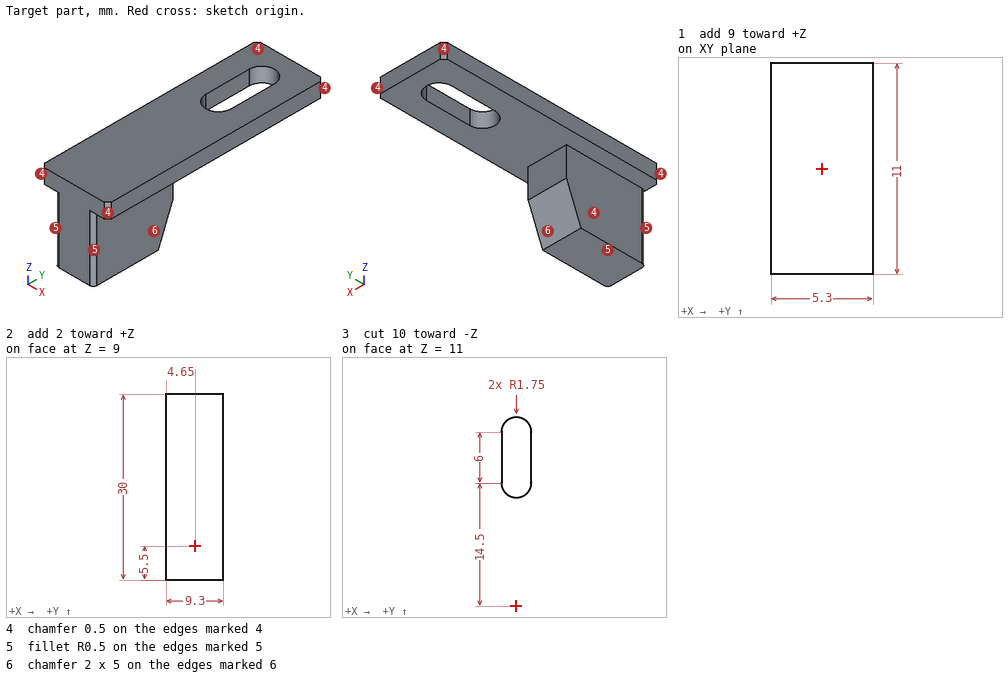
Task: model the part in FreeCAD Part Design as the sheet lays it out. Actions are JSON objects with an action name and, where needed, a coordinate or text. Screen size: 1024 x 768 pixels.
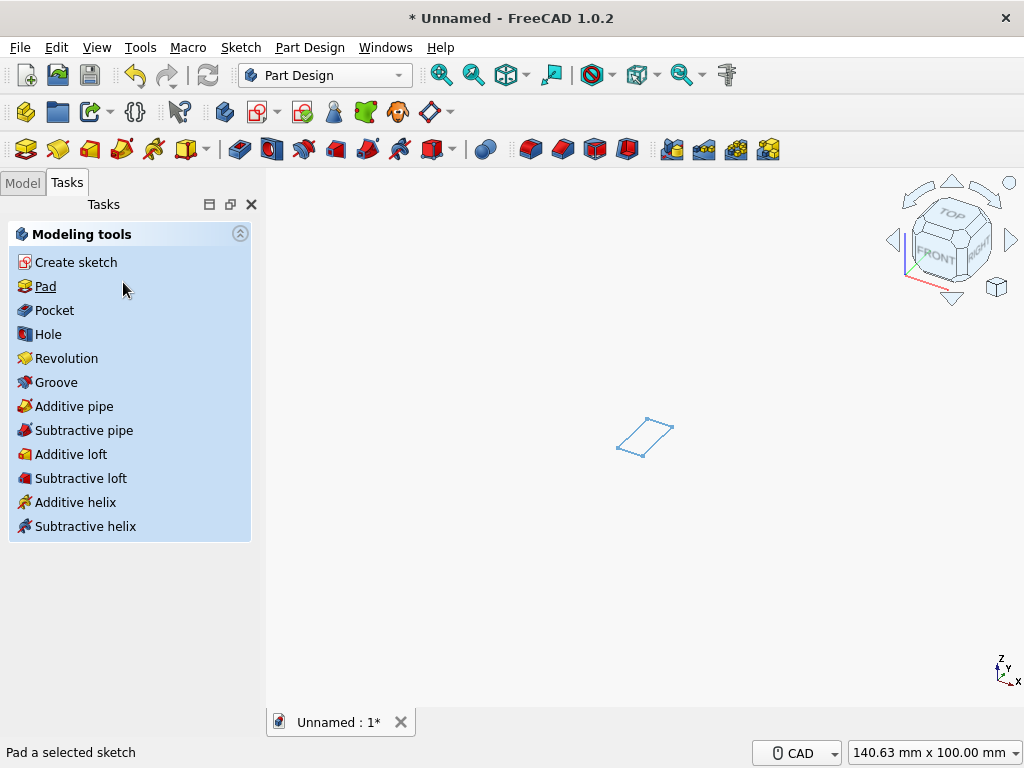
{"action": "left_click", "coordinate": [26, 150]}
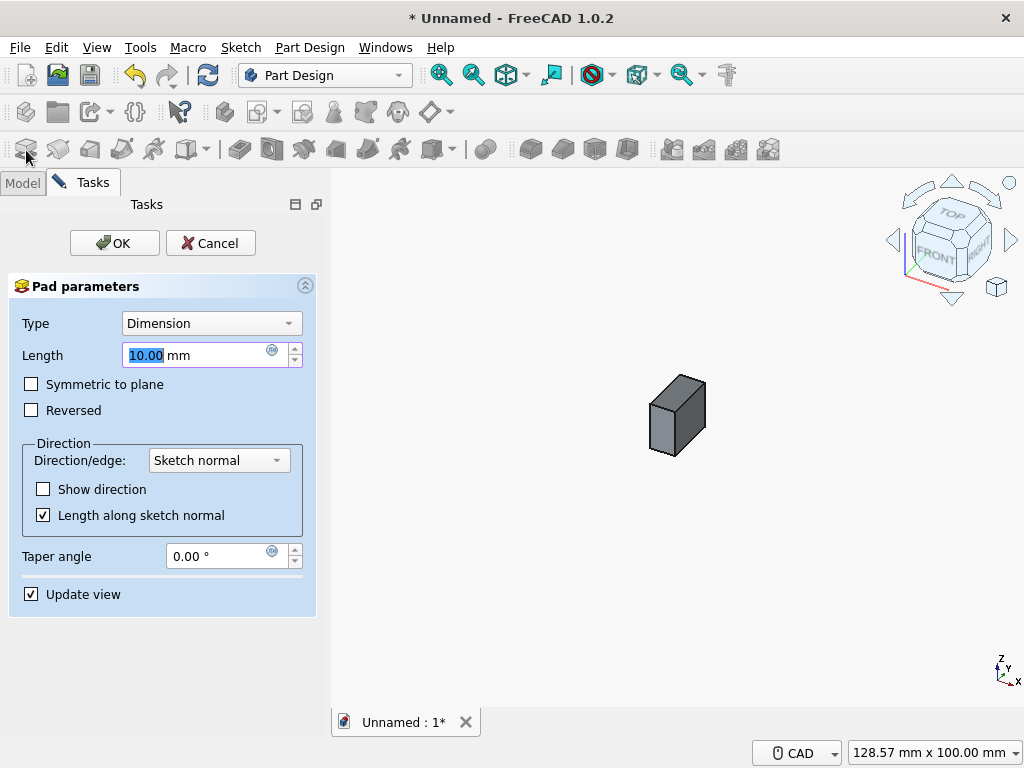
{"action": "type", "text": "9"}
{"action": "key", "text": "Tab"}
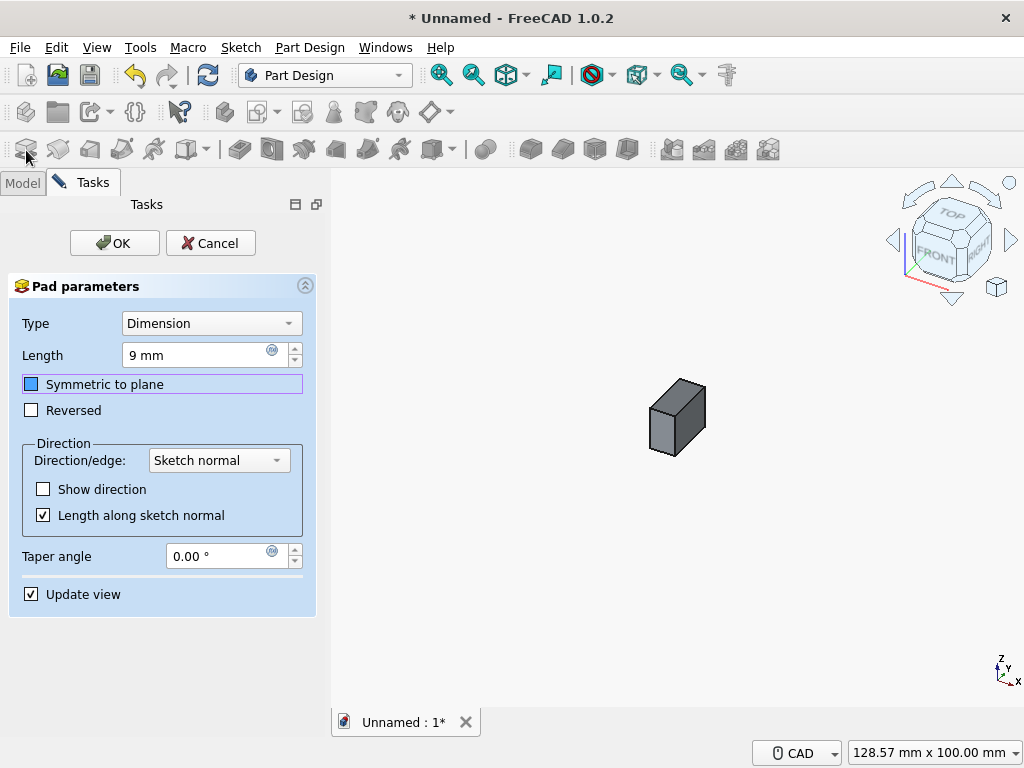
{"action": "left_click", "coordinate": [115, 243]}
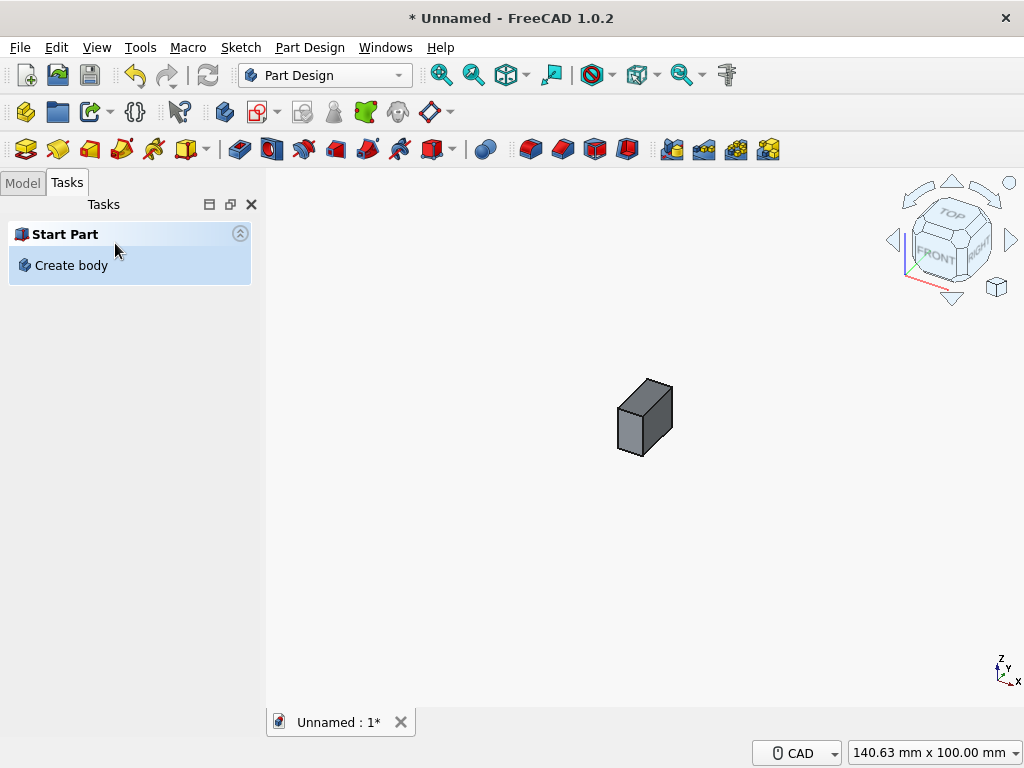
{"action": "left_click", "coordinate": [442, 76]}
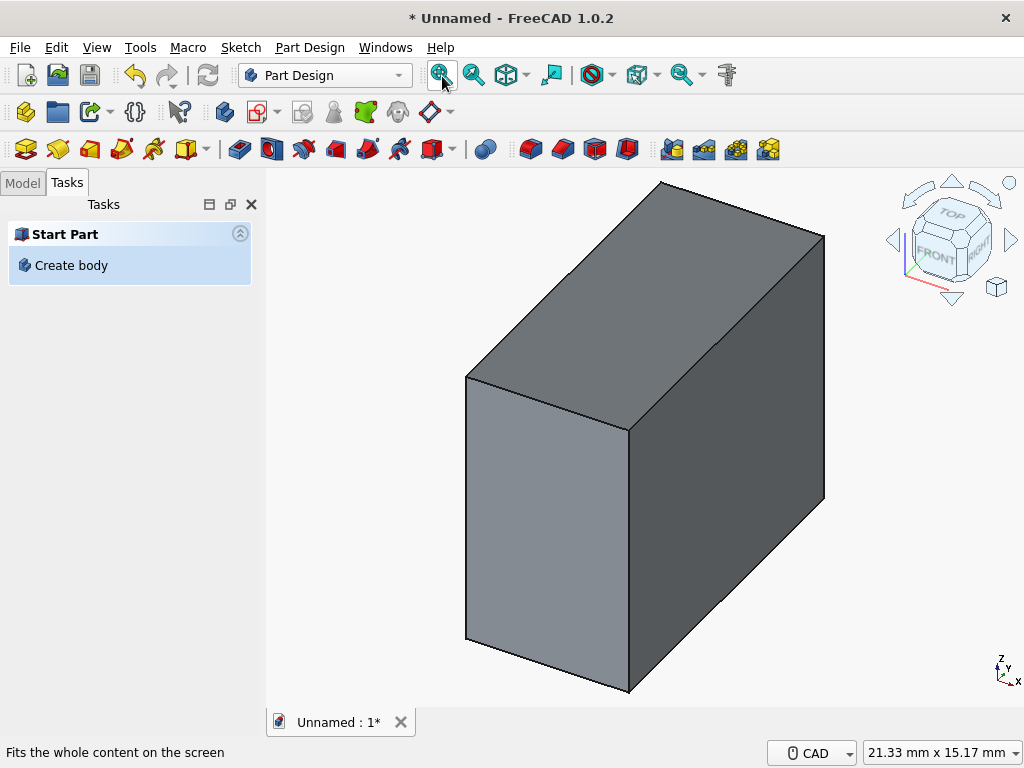
{"action": "left_click", "coordinate": [673, 278]}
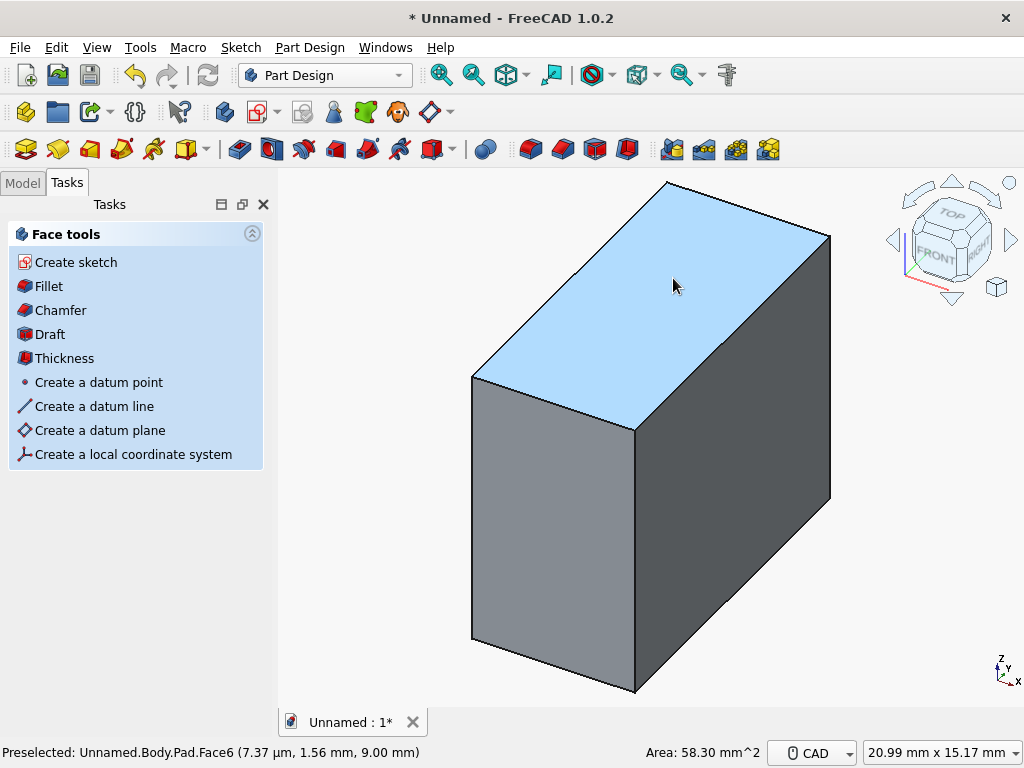
{"action": "left_click", "coordinate": [258, 112]}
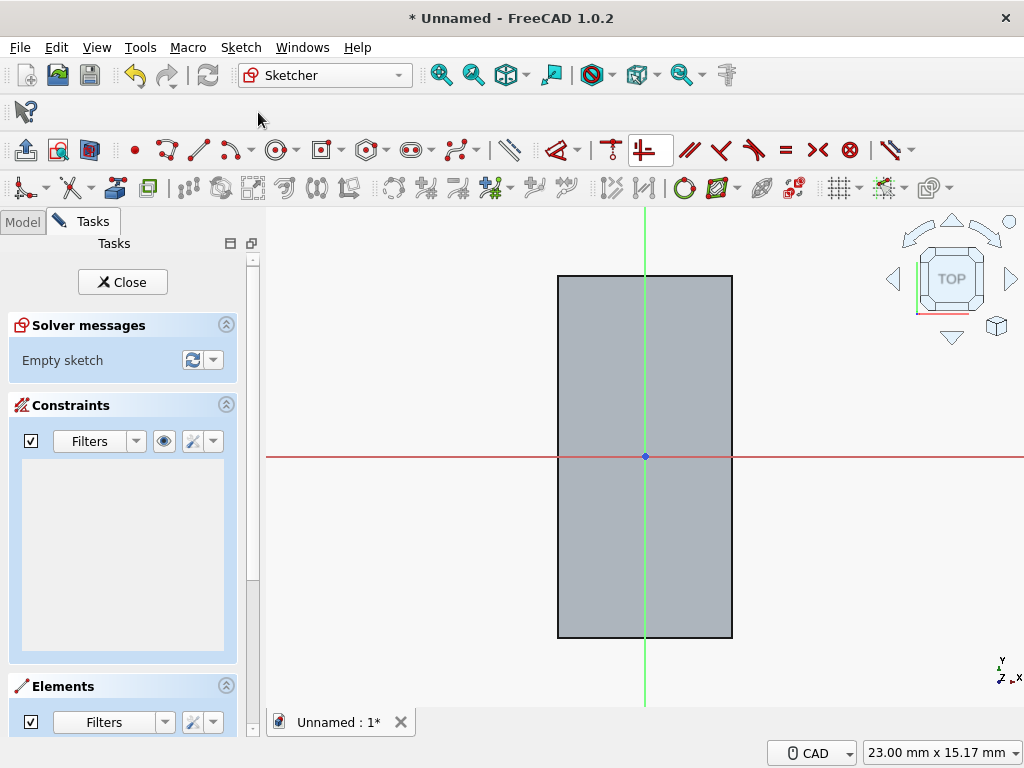
{"action": "scroll", "coordinate": [547, 592], "scroll_direction": "down", "scroll_amount": 6}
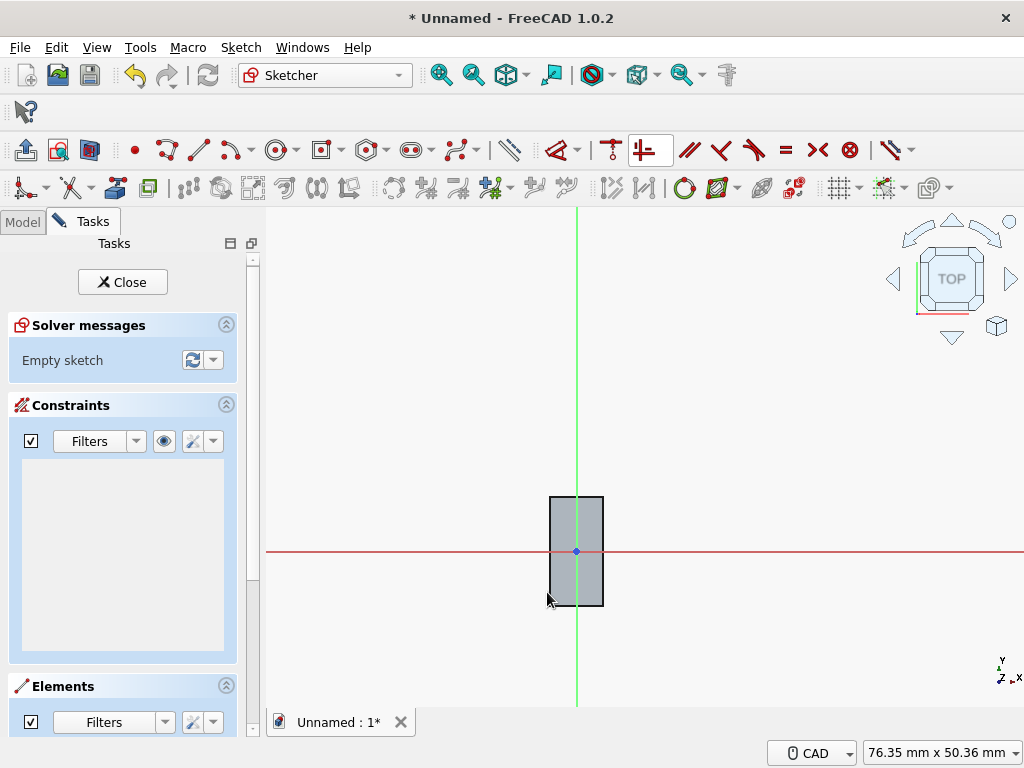
{"action": "key", "text": "g r"}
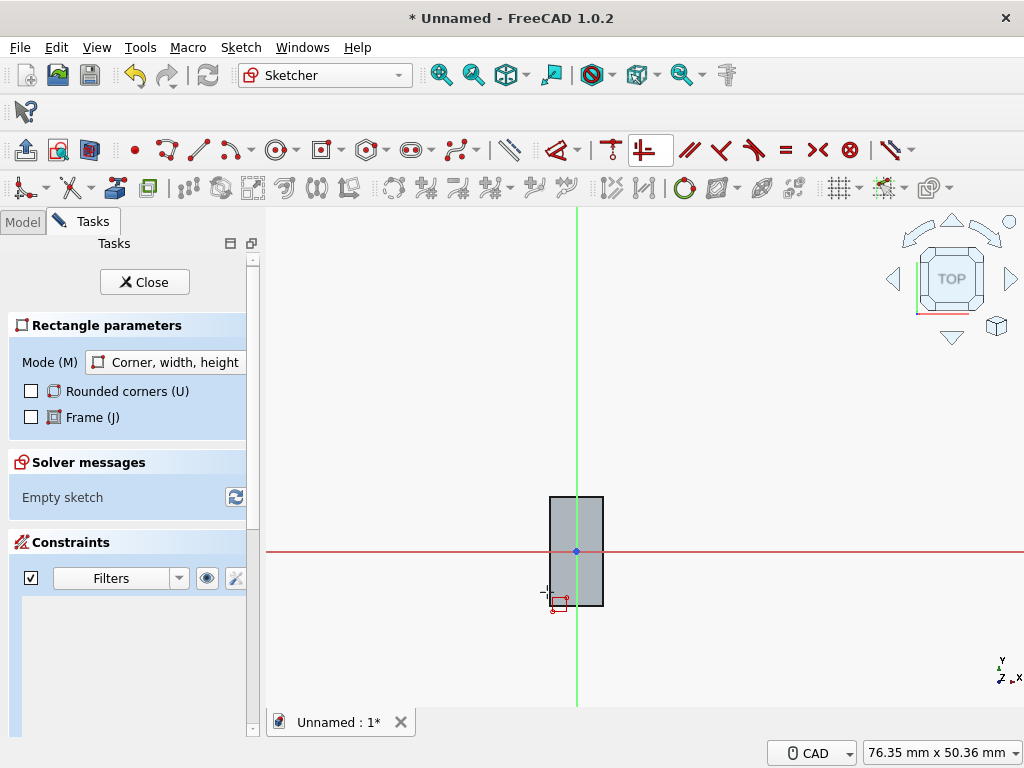
{"action": "left_click", "coordinate": [531, 309]}
{"action": "left_click", "coordinate": [623, 606]}
{"action": "key", "text": "Escape"}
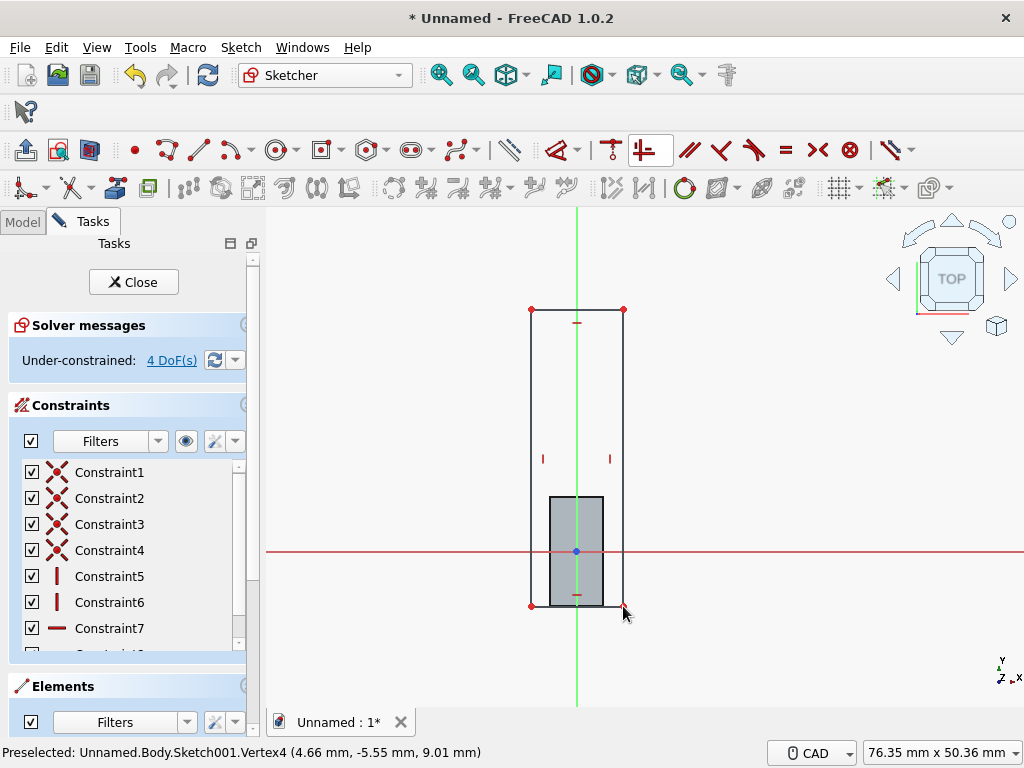
{"action": "left_click", "coordinate": [556, 150]}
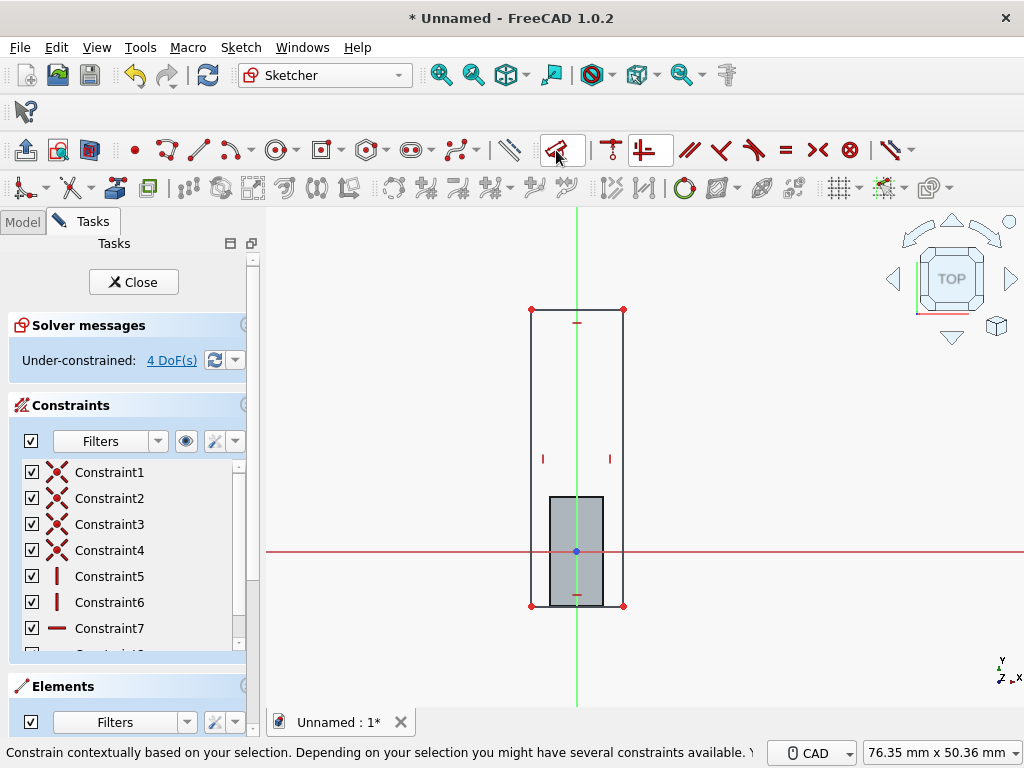
{"action": "left_click", "coordinate": [531, 399]}
{"action": "left_click", "coordinate": [497, 458]}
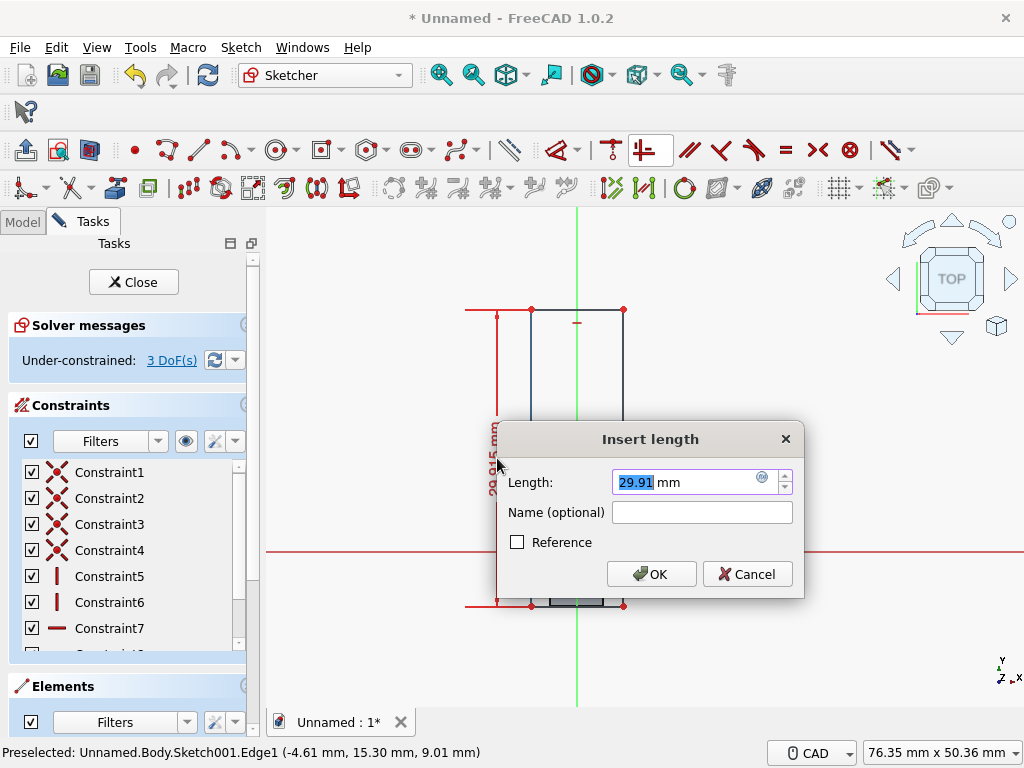
{"action": "type", "text": "30"}
{"action": "key", "text": "Return"}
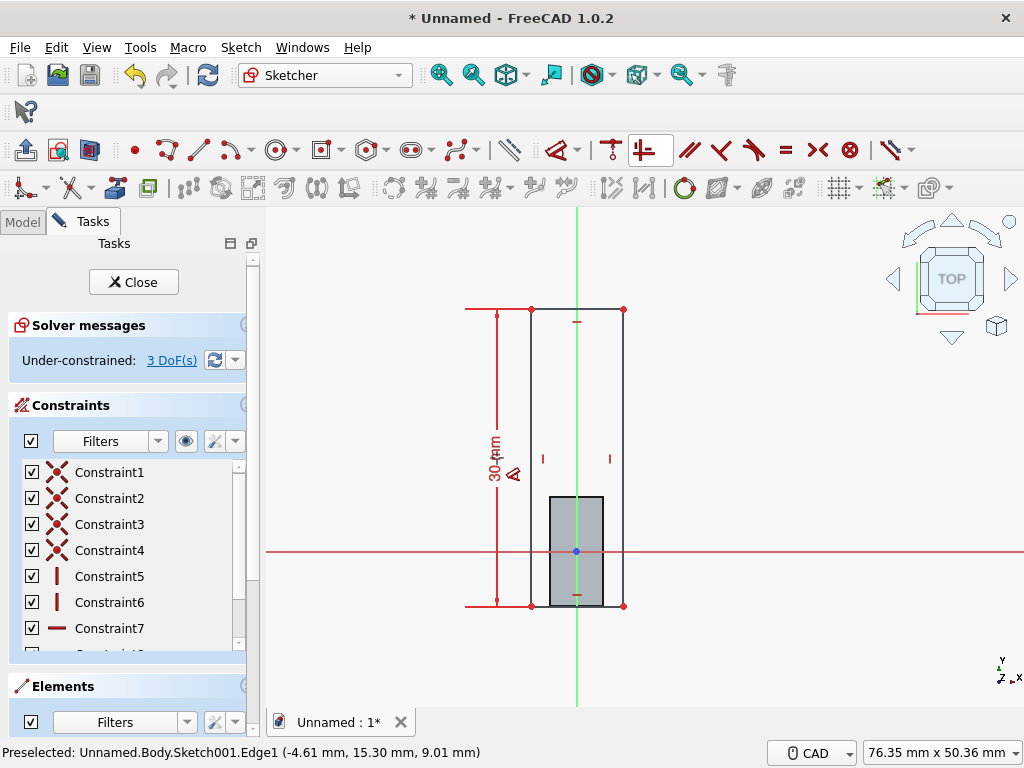
{"action": "left_click", "coordinate": [559, 607]}
{"action": "left_click", "coordinate": [556, 641]}